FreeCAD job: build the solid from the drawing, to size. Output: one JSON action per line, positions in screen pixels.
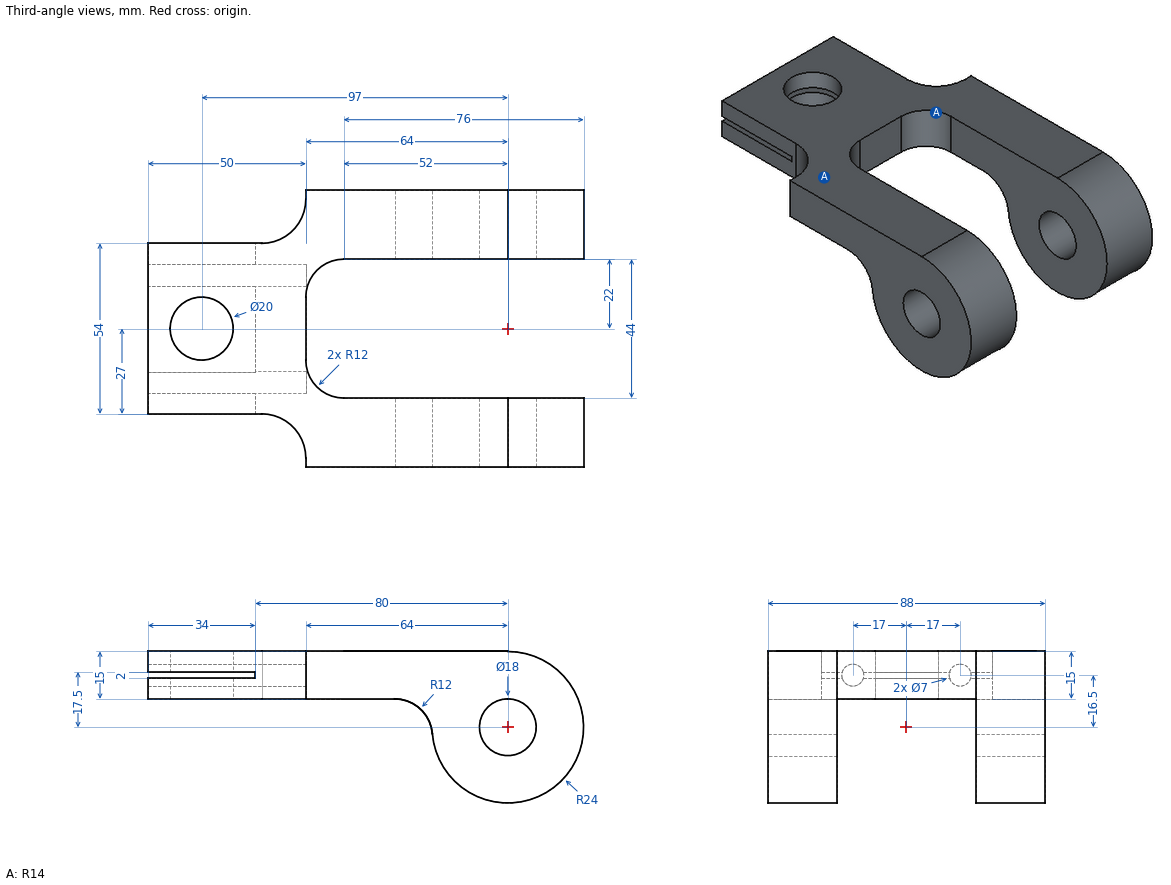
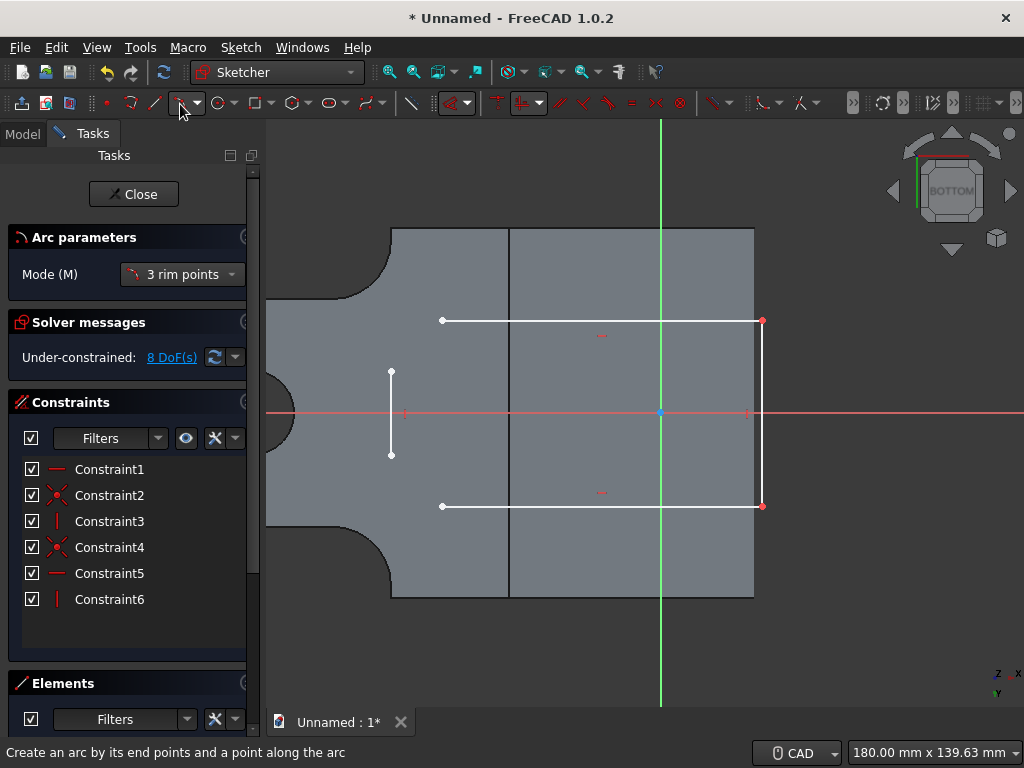
{"action": "left_click", "coordinate": [442, 321]}
{"action": "left_click", "coordinate": [391, 372]}
{"action": "left_click", "coordinate": [406, 335]}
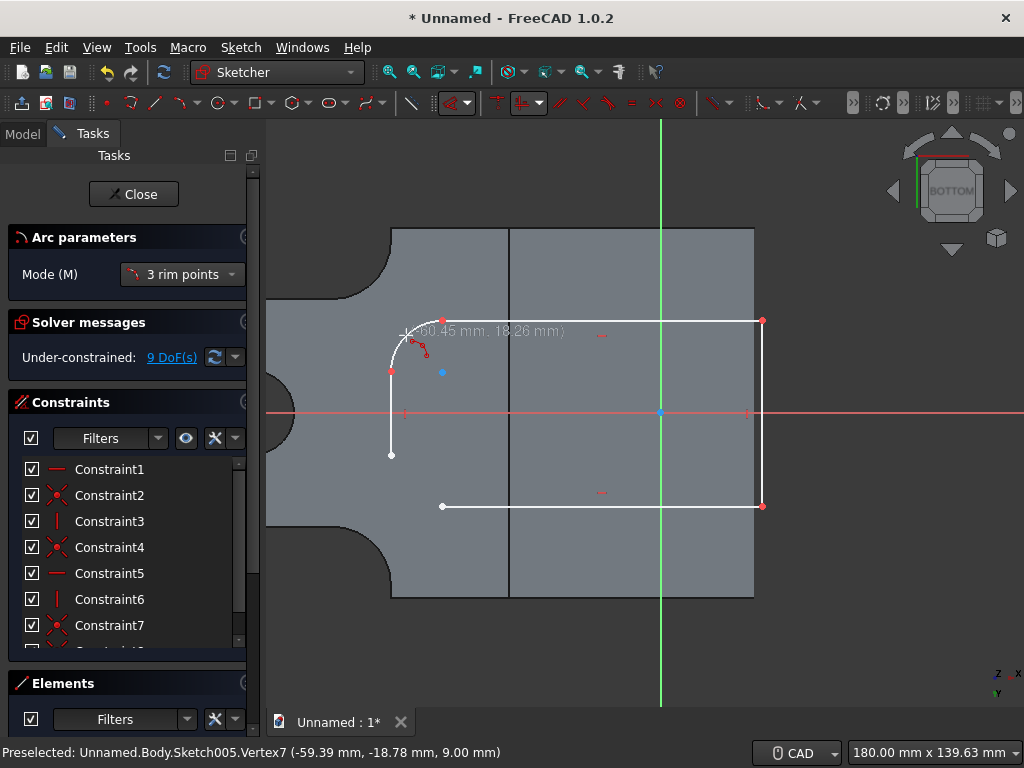
{"action": "left_click", "coordinate": [391, 456]}
{"action": "left_click", "coordinate": [442, 507]}
{"action": "left_click", "coordinate": [406, 491]}
{"action": "key", "text": "Escape"}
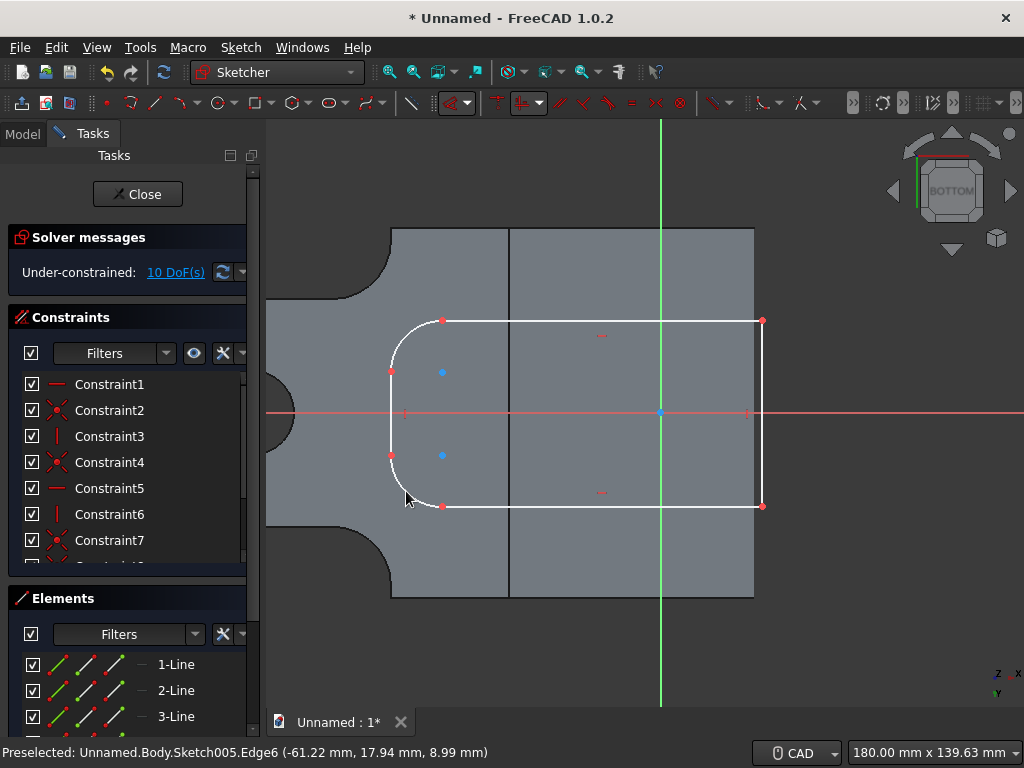
{"action": "left_click", "coordinate": [538, 507]}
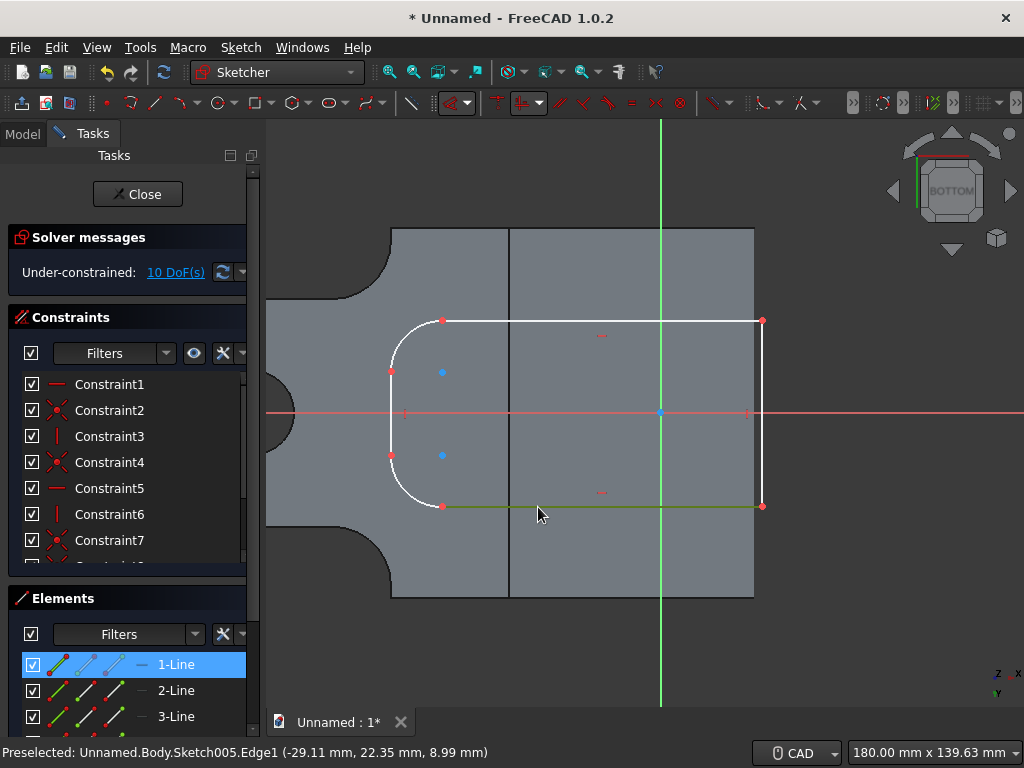
{"action": "left_click", "coordinate": [397, 479]}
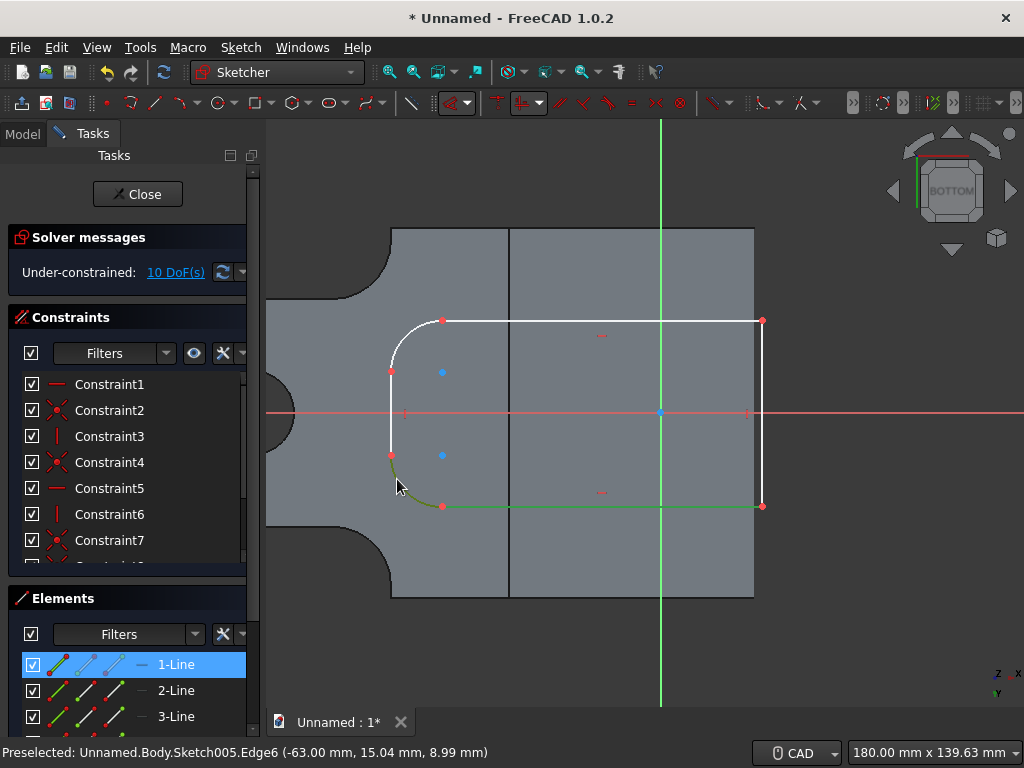
{"action": "left_click", "coordinate": [608, 104]}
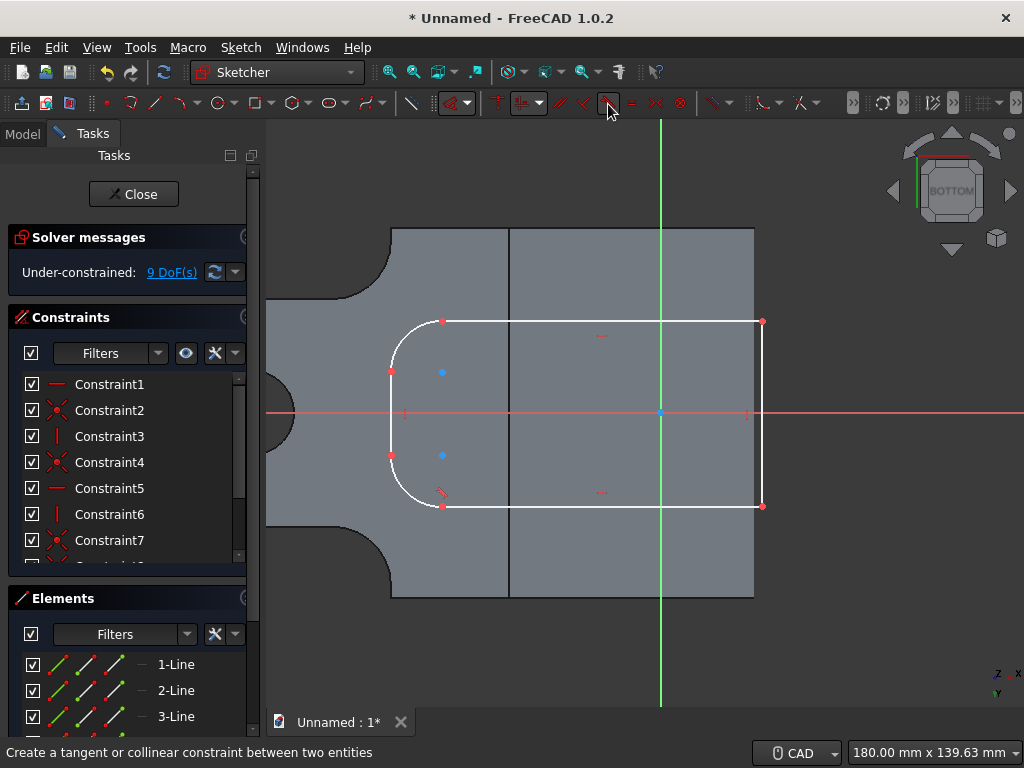
{"action": "left_click", "coordinate": [538, 321]}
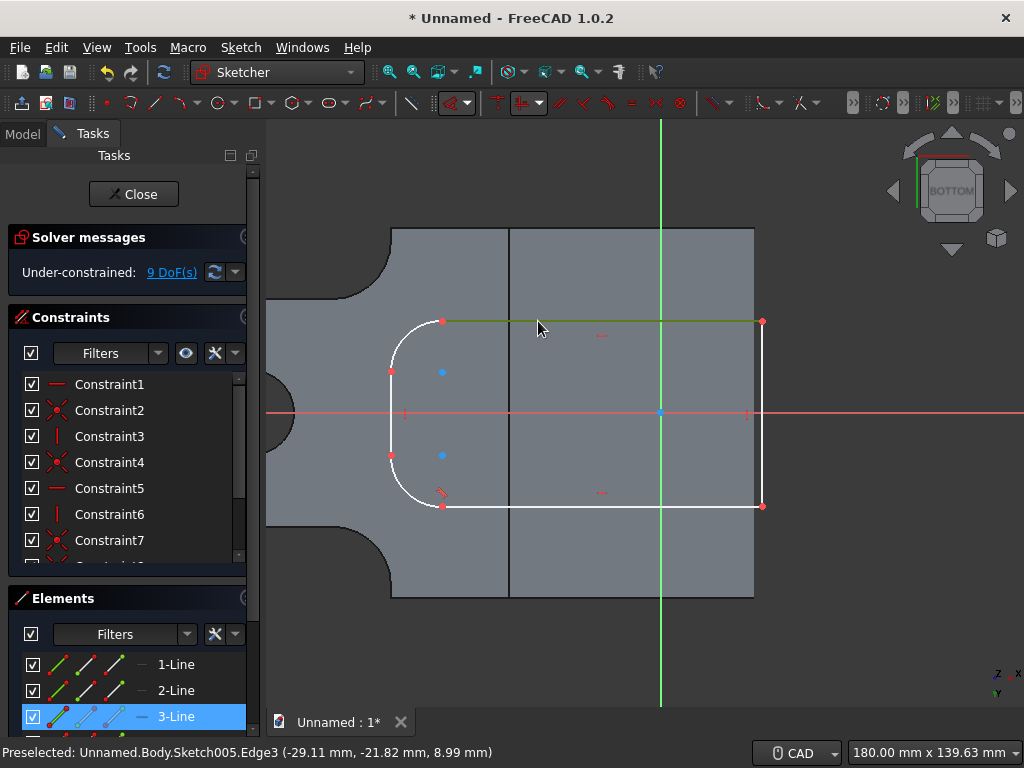
{"action": "left_click", "coordinate": [419, 327]}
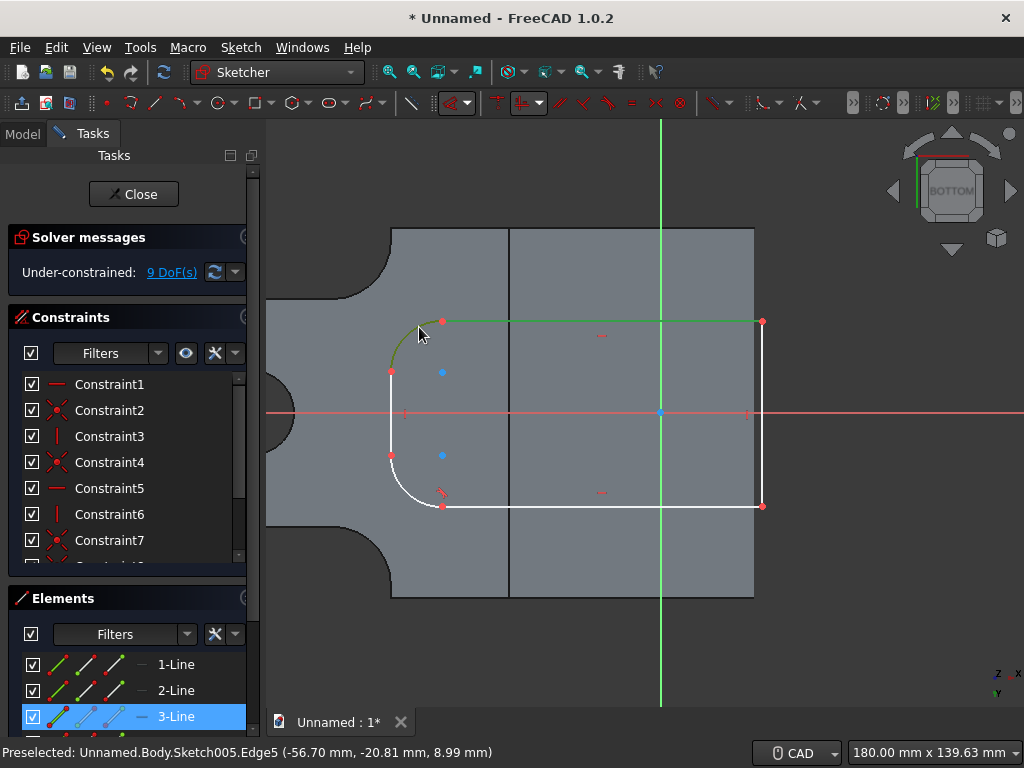
{"action": "left_click", "coordinate": [608, 104]}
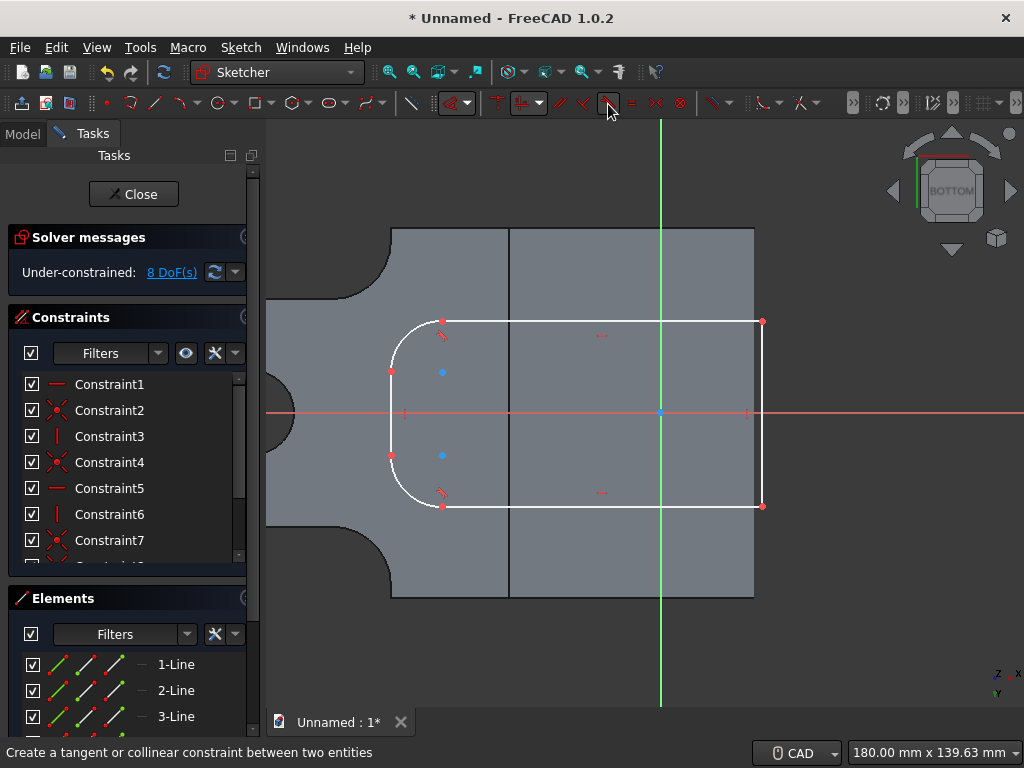
{"action": "left_click", "coordinate": [391, 397]}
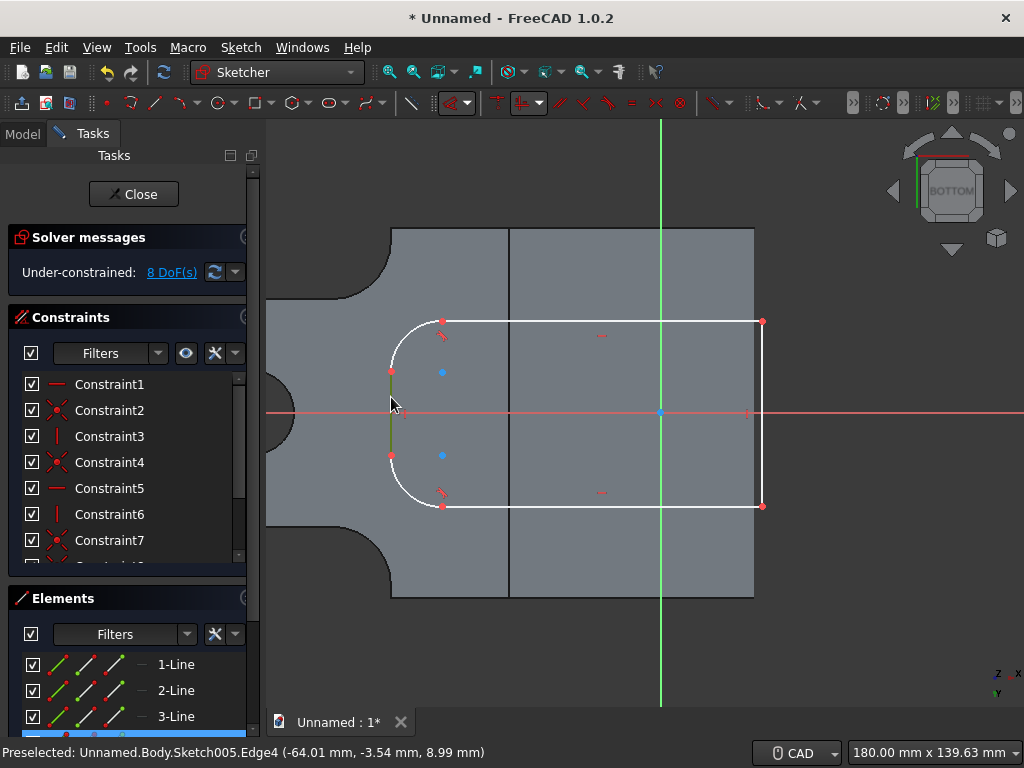
{"action": "left_click", "coordinate": [419, 327]}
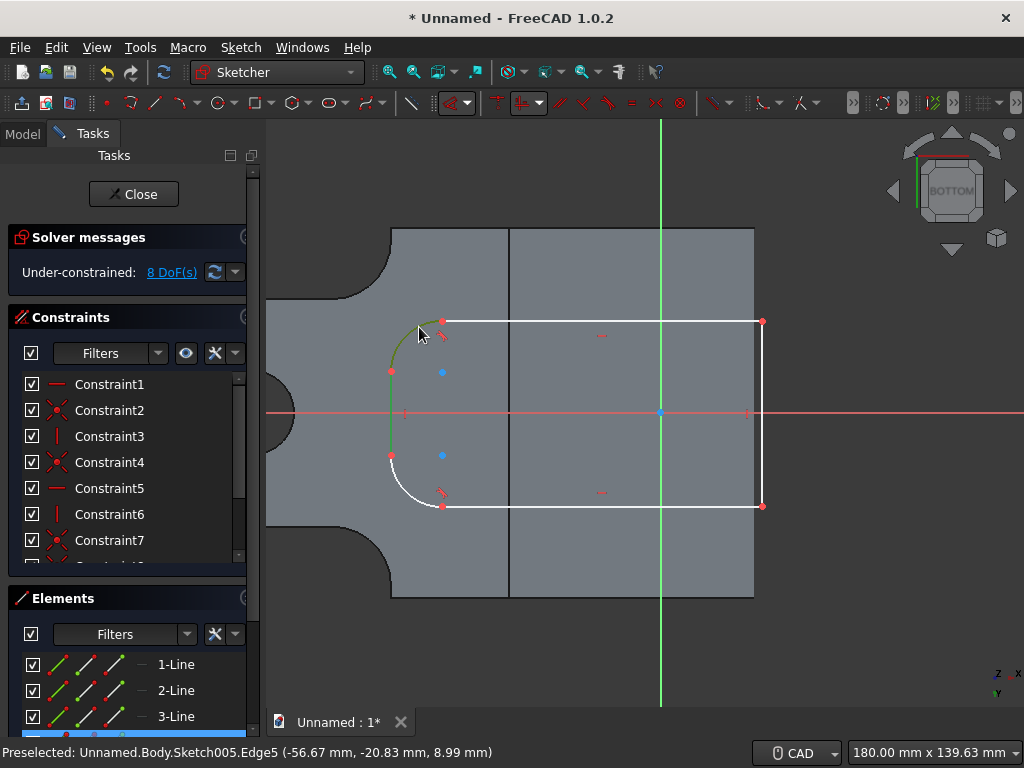
{"action": "left_click", "coordinate": [608, 104]}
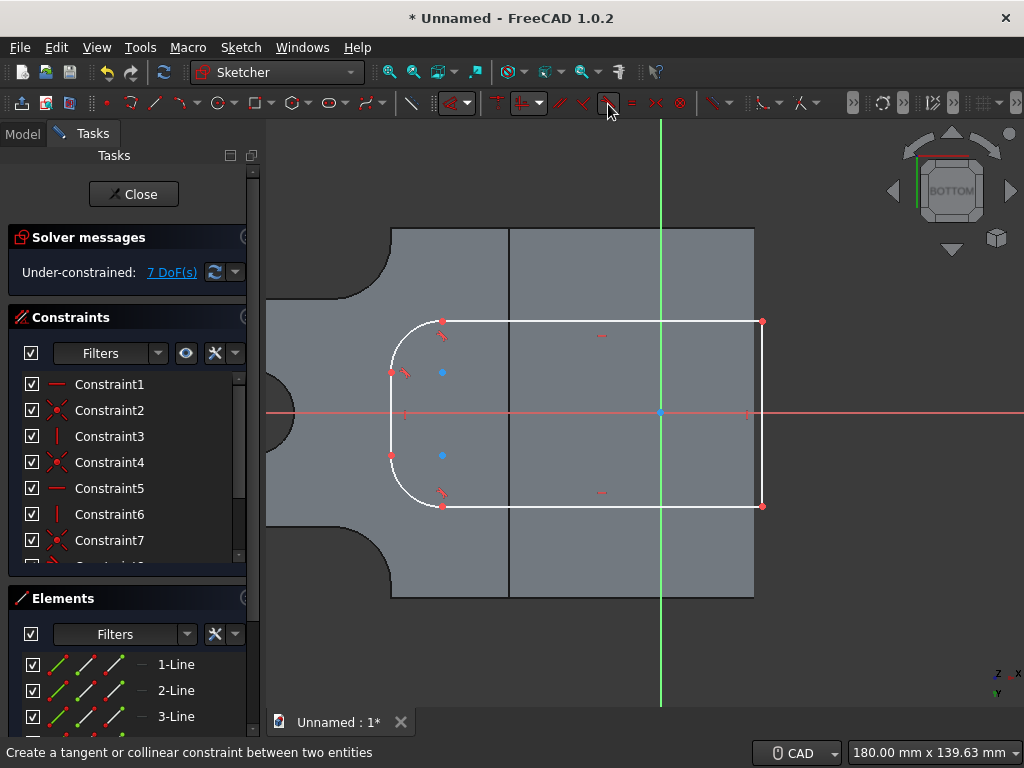
{"action": "left_click", "coordinate": [391, 397]}